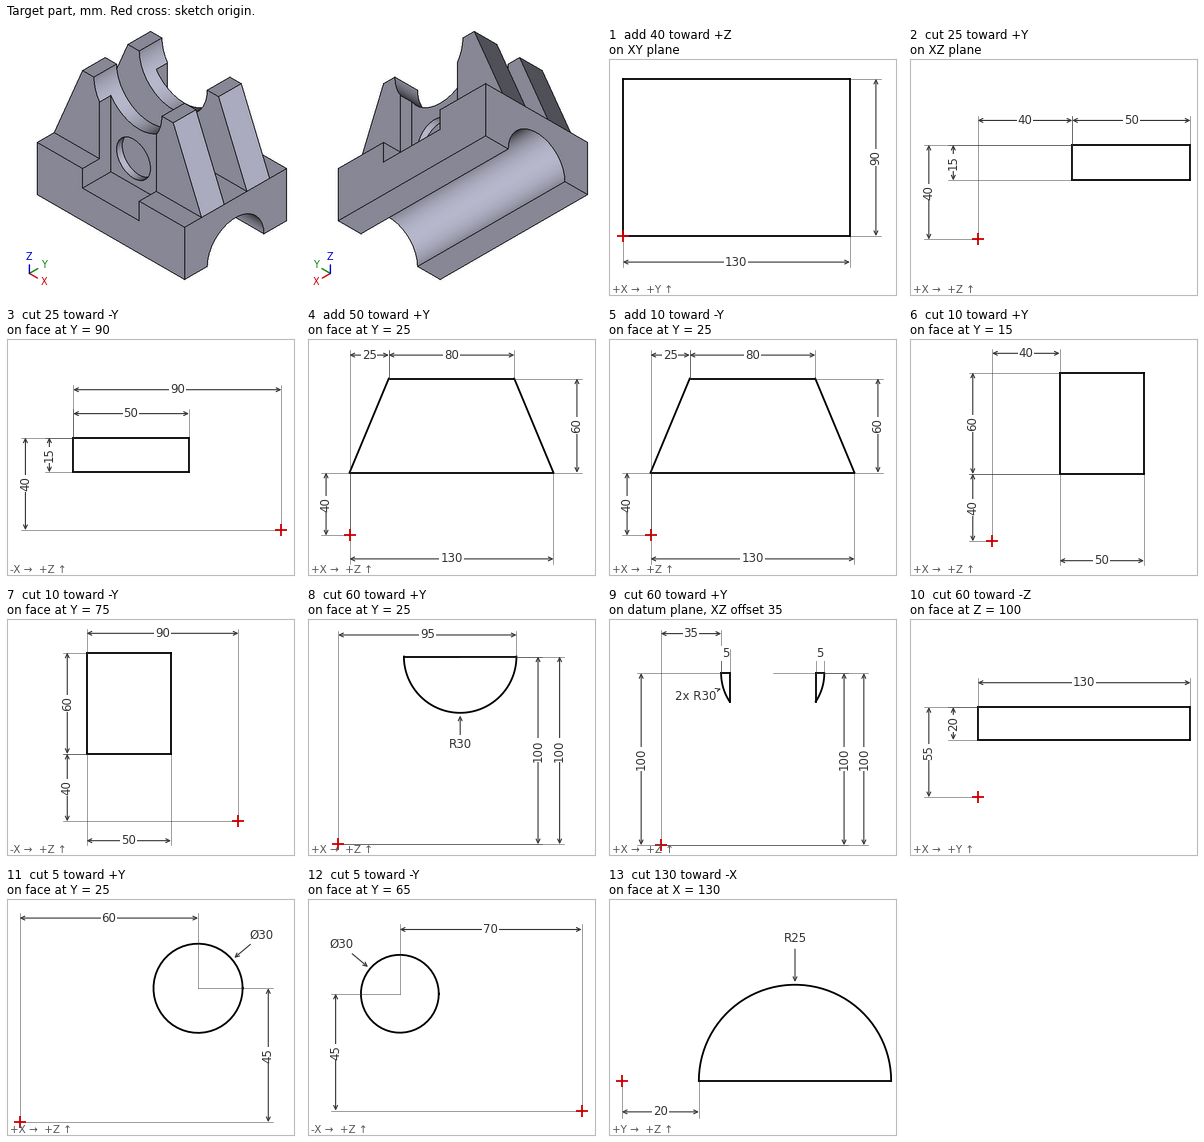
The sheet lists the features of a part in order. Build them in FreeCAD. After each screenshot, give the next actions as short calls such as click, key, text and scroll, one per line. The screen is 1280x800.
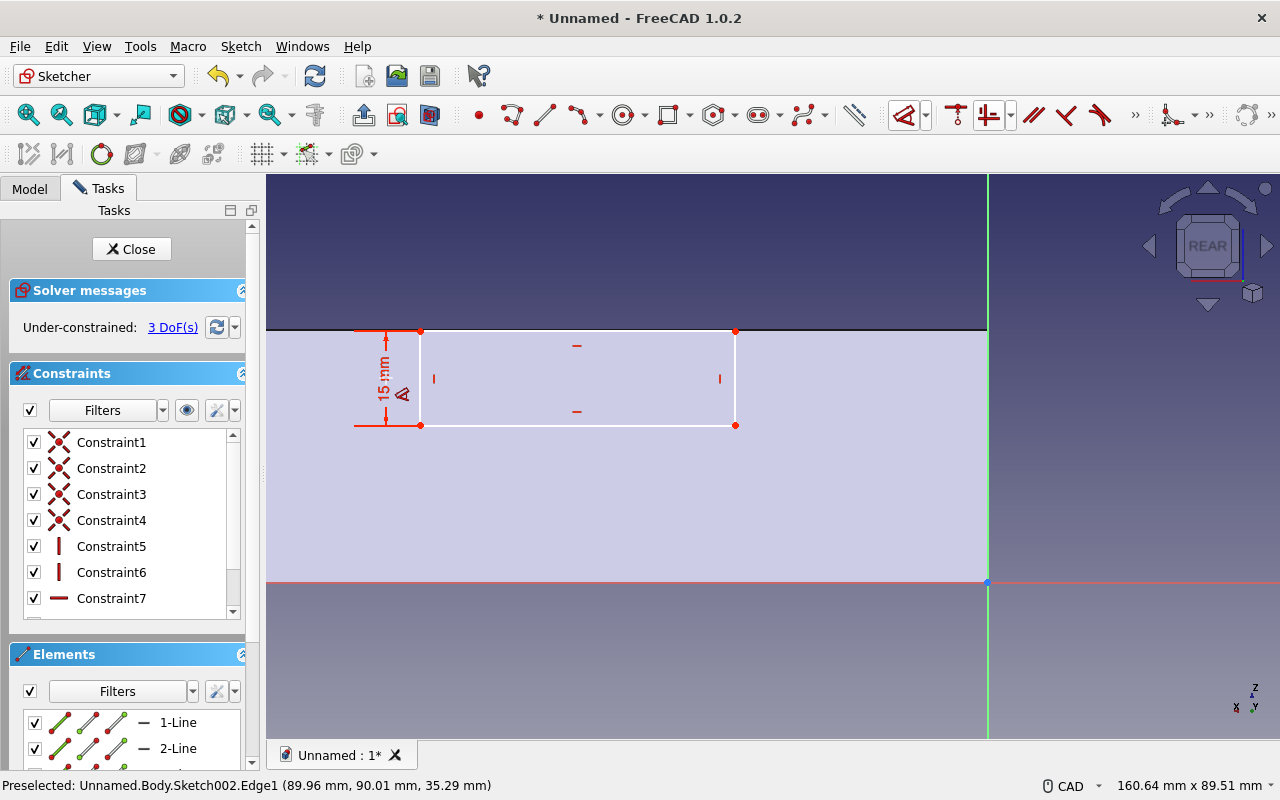
click(515, 426)
click(578, 392)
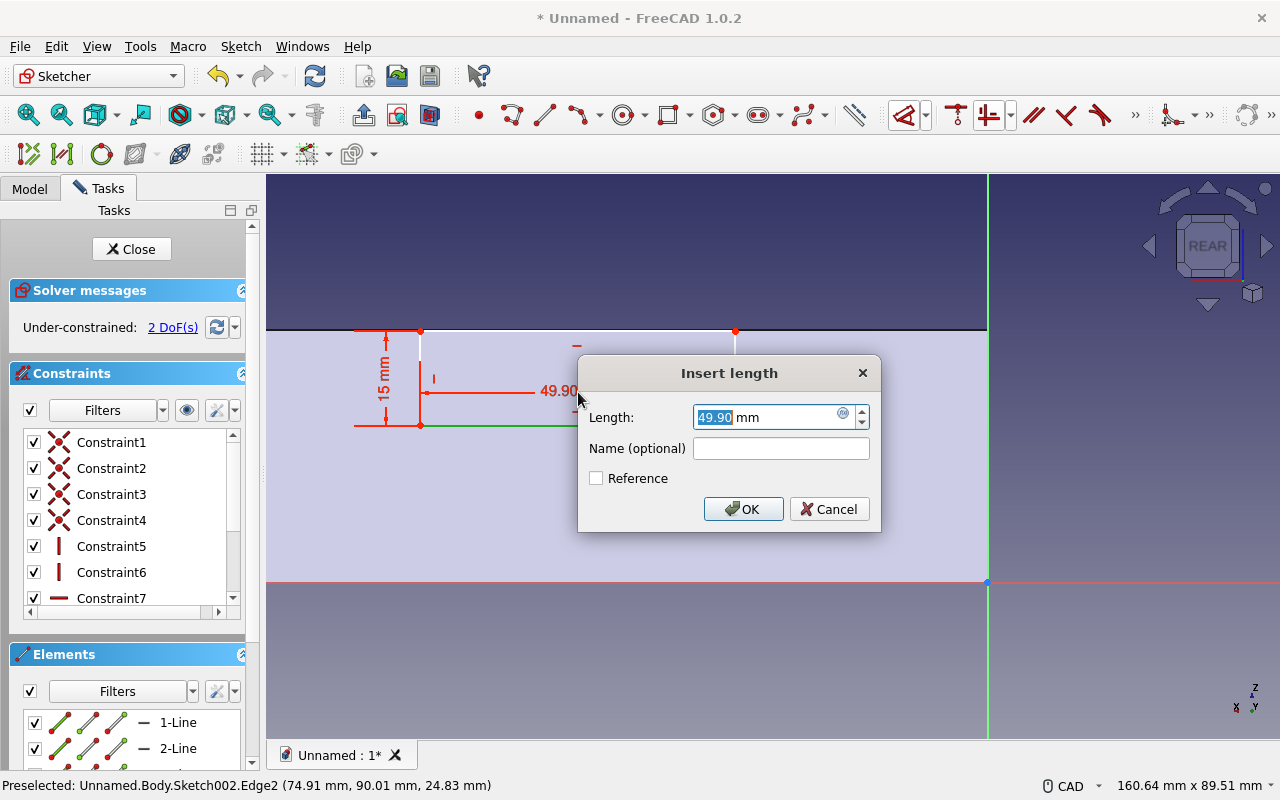
text(50)
key(Return)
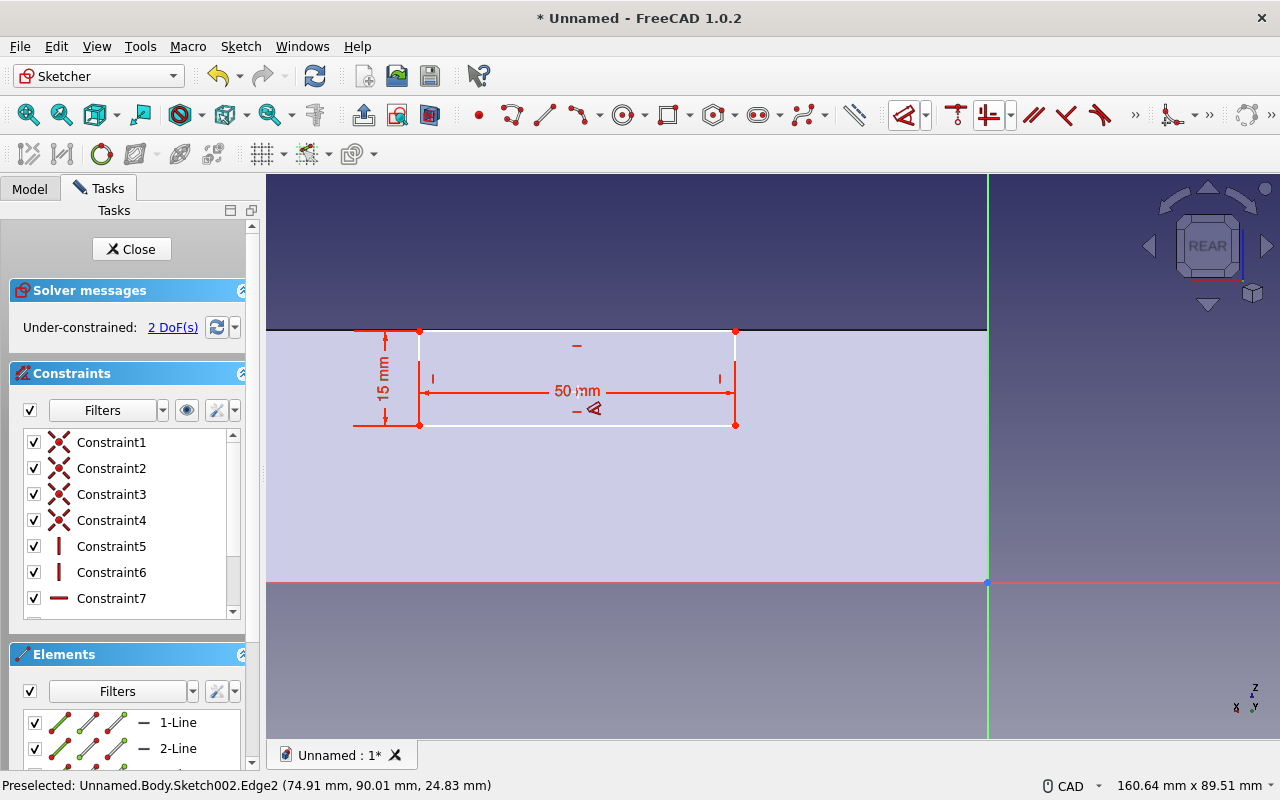
click(419, 331)
click(704, 617)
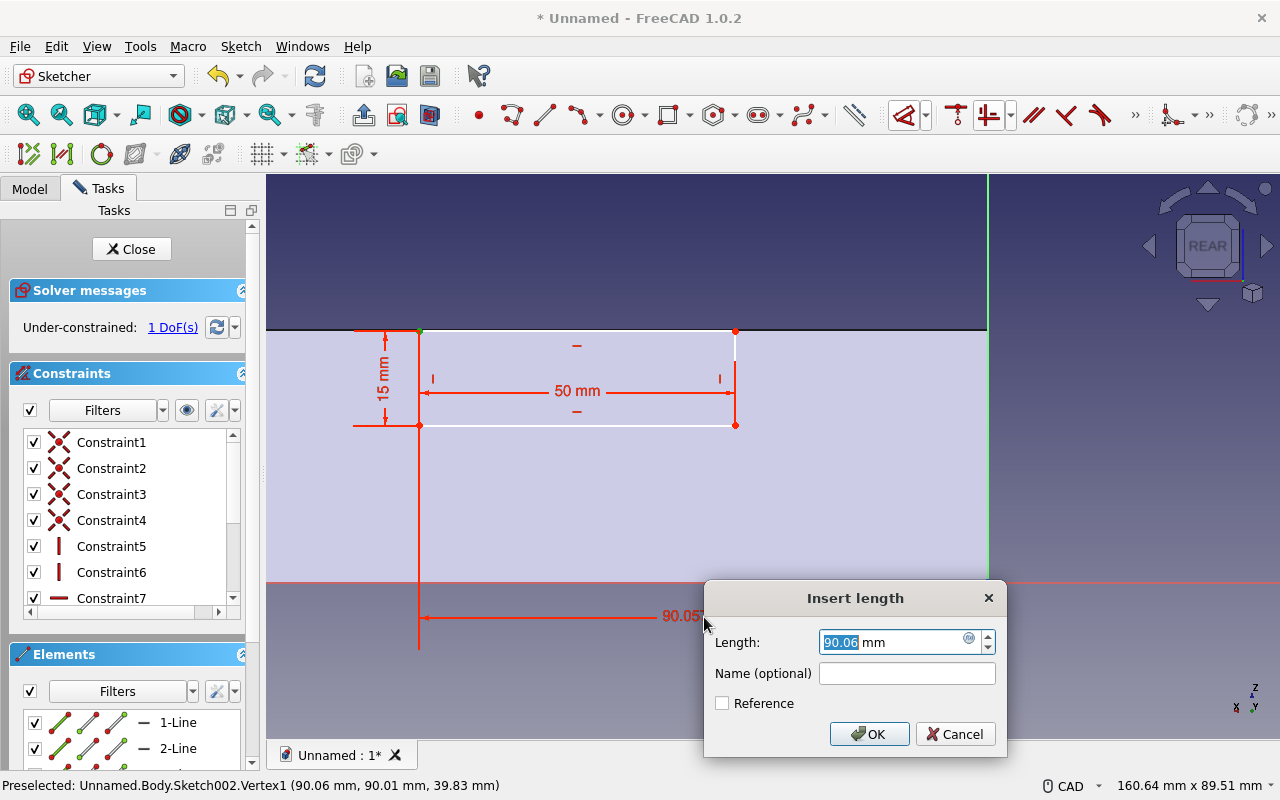
text(90)
key(Return)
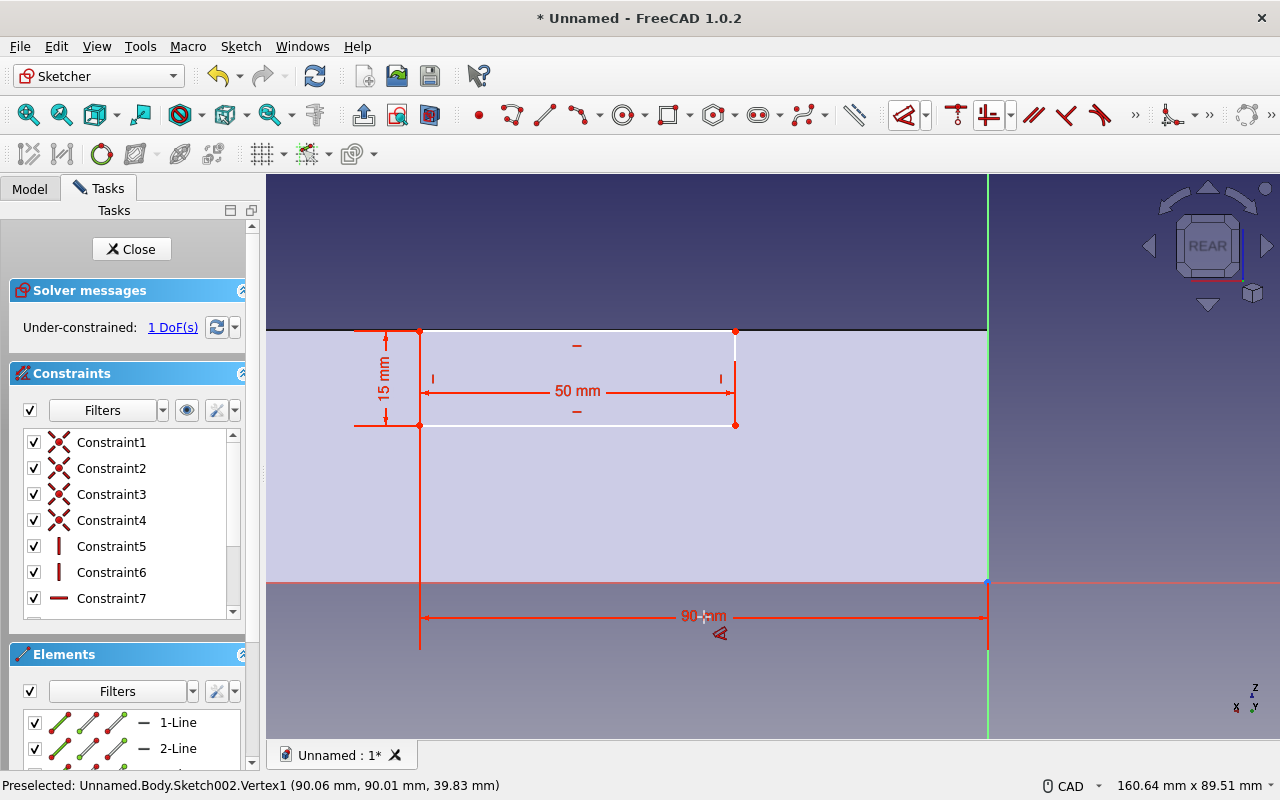
click(420, 331)
click(1022, 457)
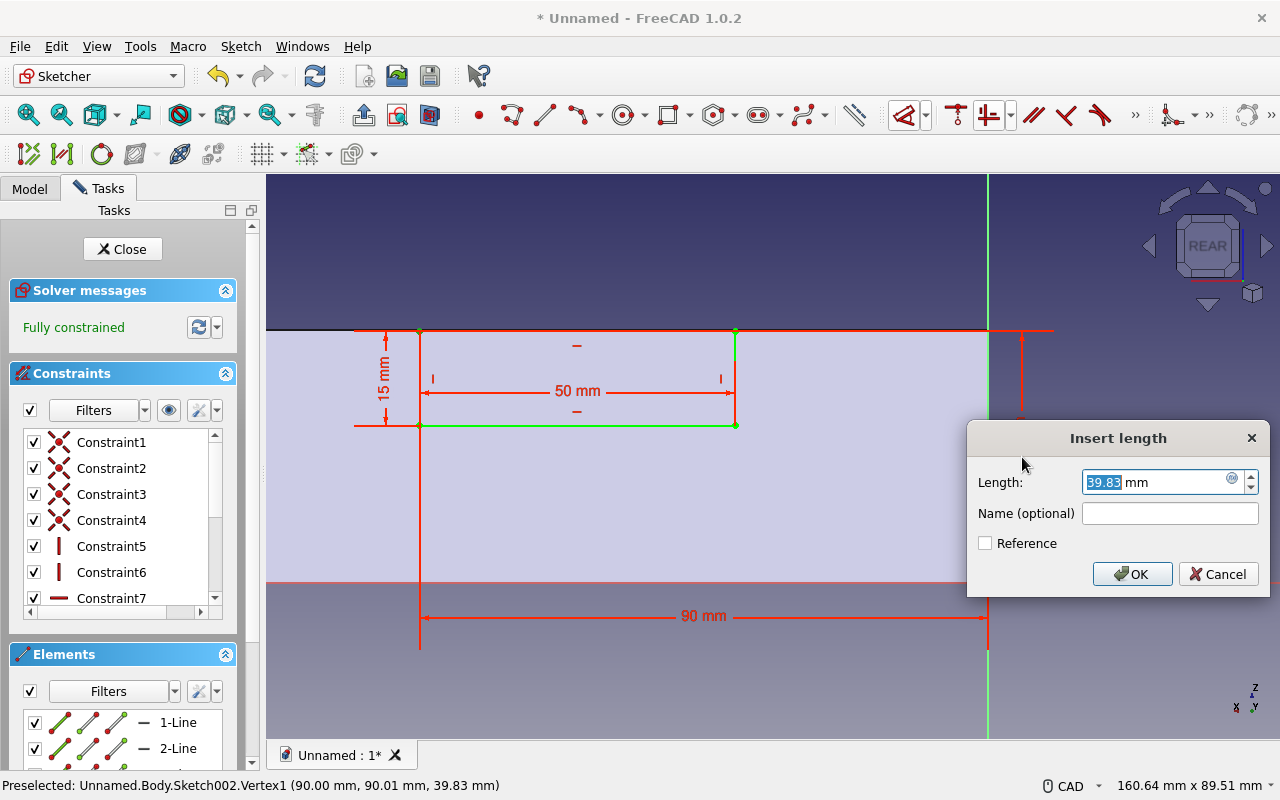
text(40)
key(Return)
key(Escape)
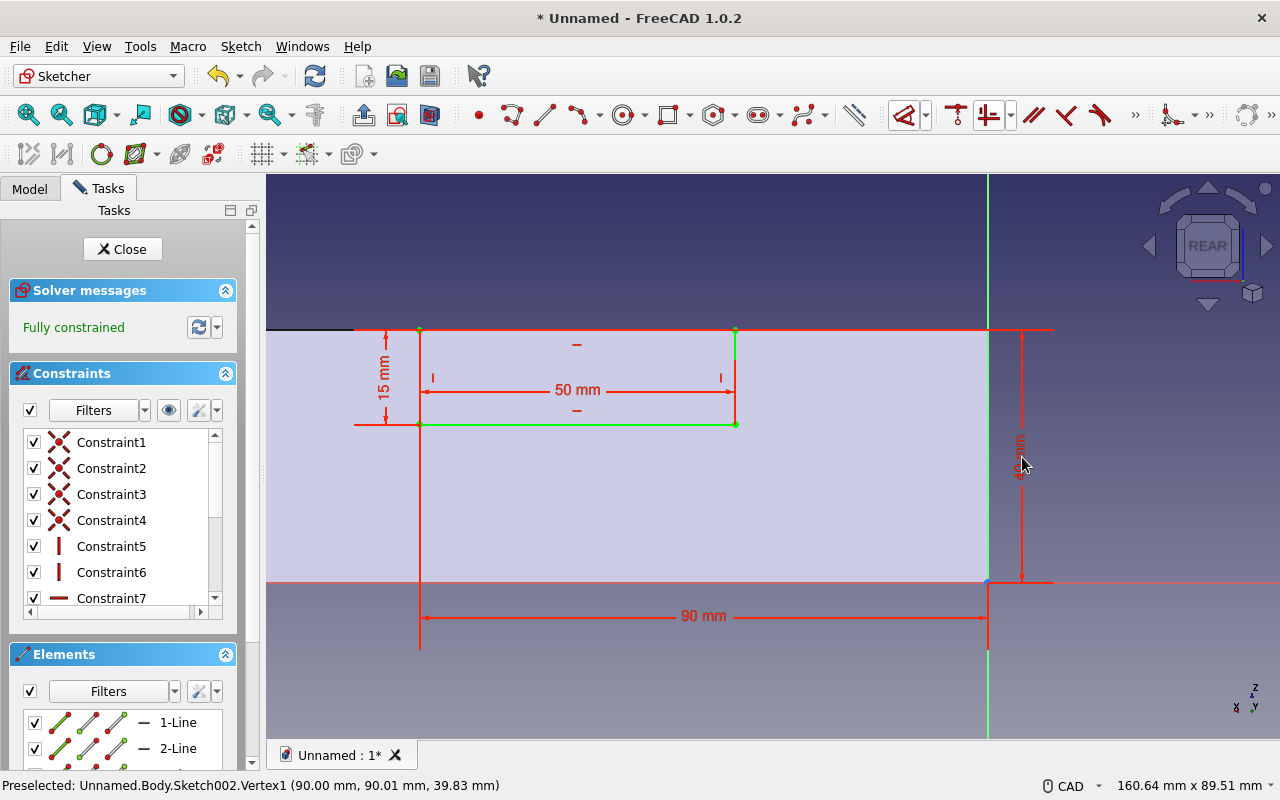
click(123, 249)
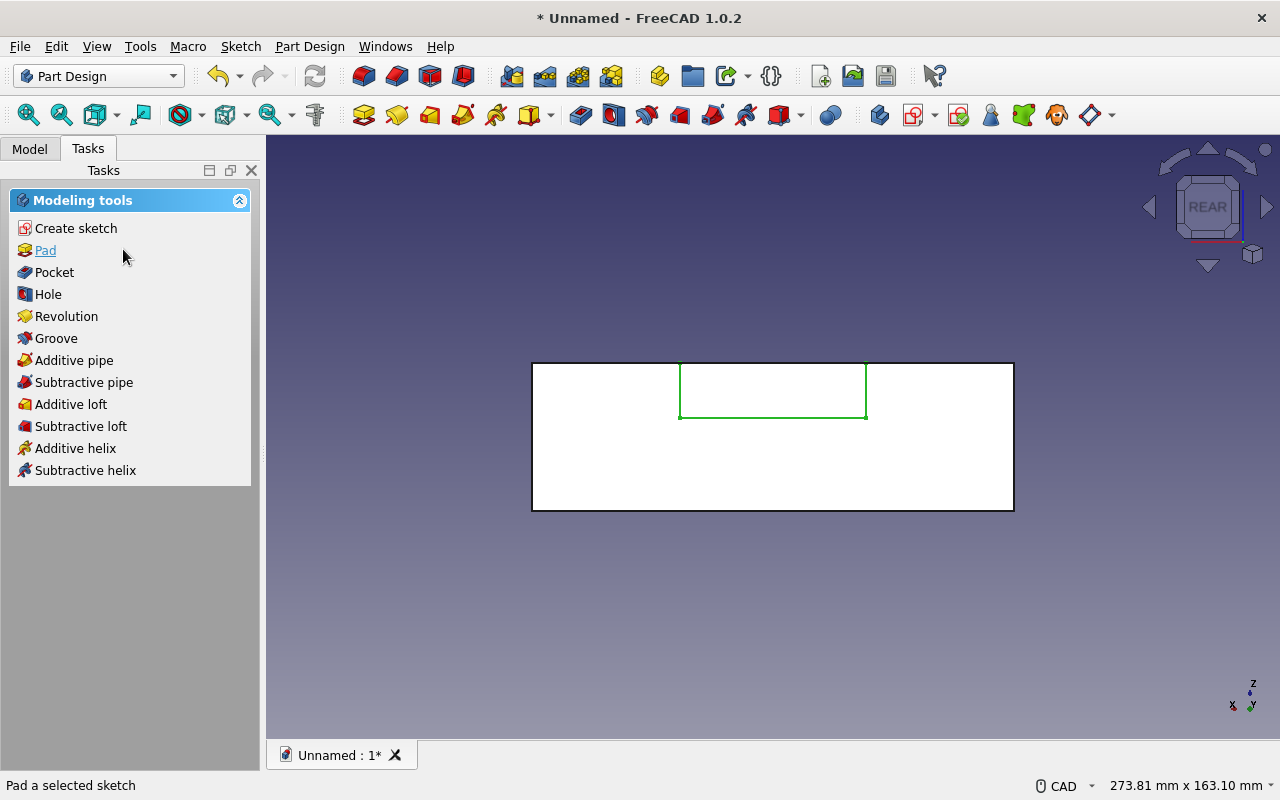
click(581, 116)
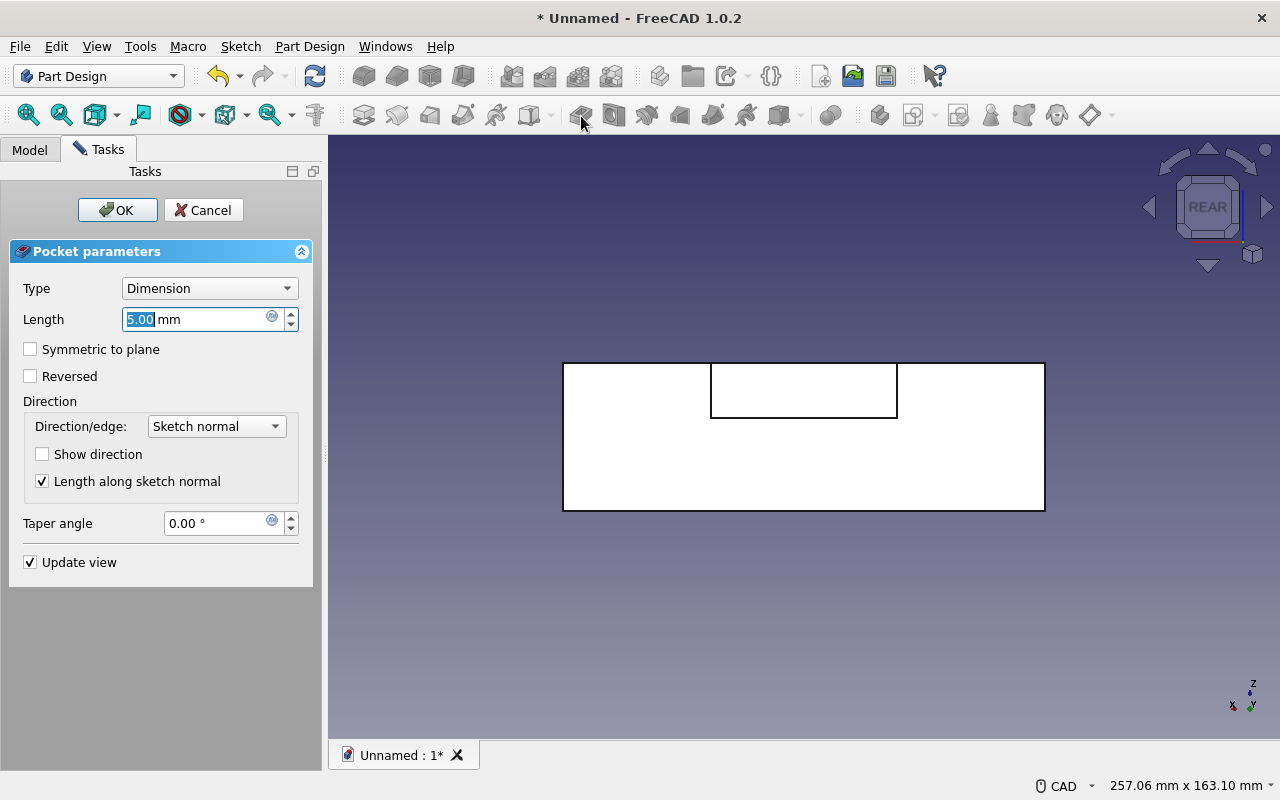
text(25)
key(Tab)